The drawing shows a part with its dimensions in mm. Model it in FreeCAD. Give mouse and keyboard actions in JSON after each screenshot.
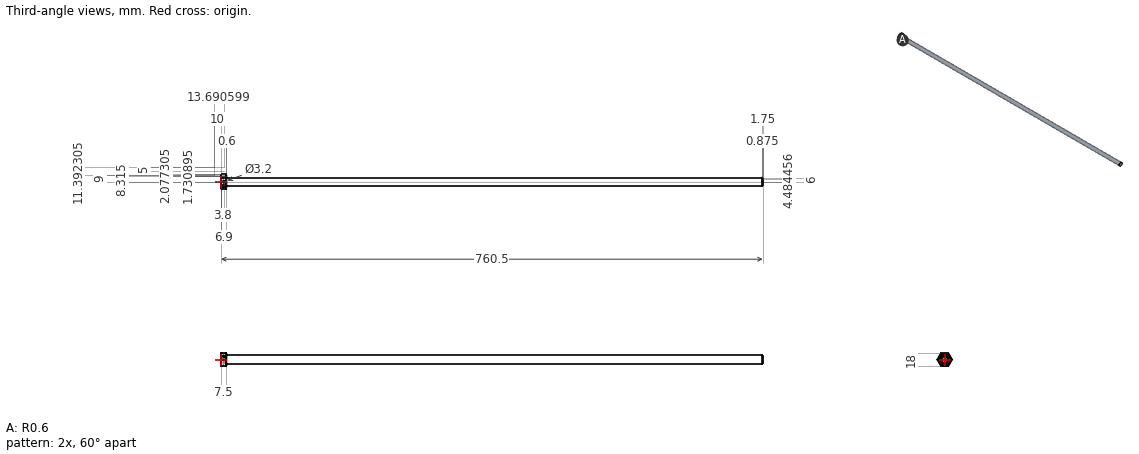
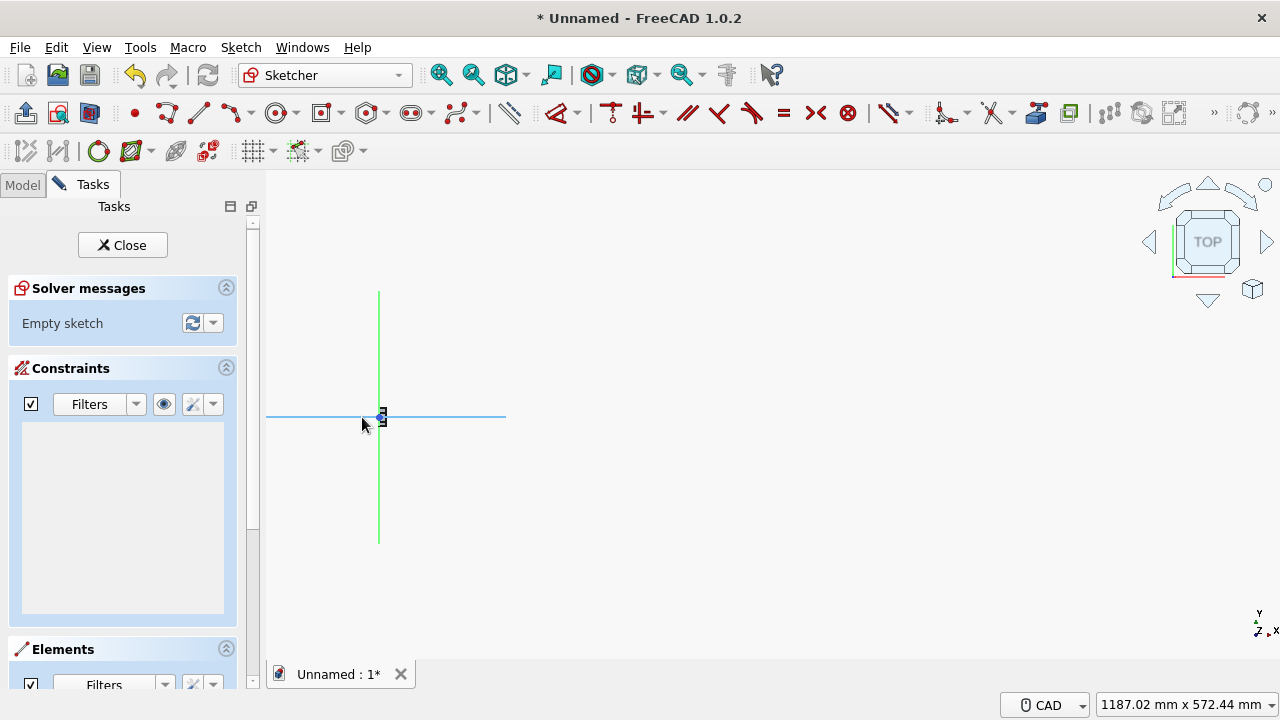
{"action": "key", "text": "g r"}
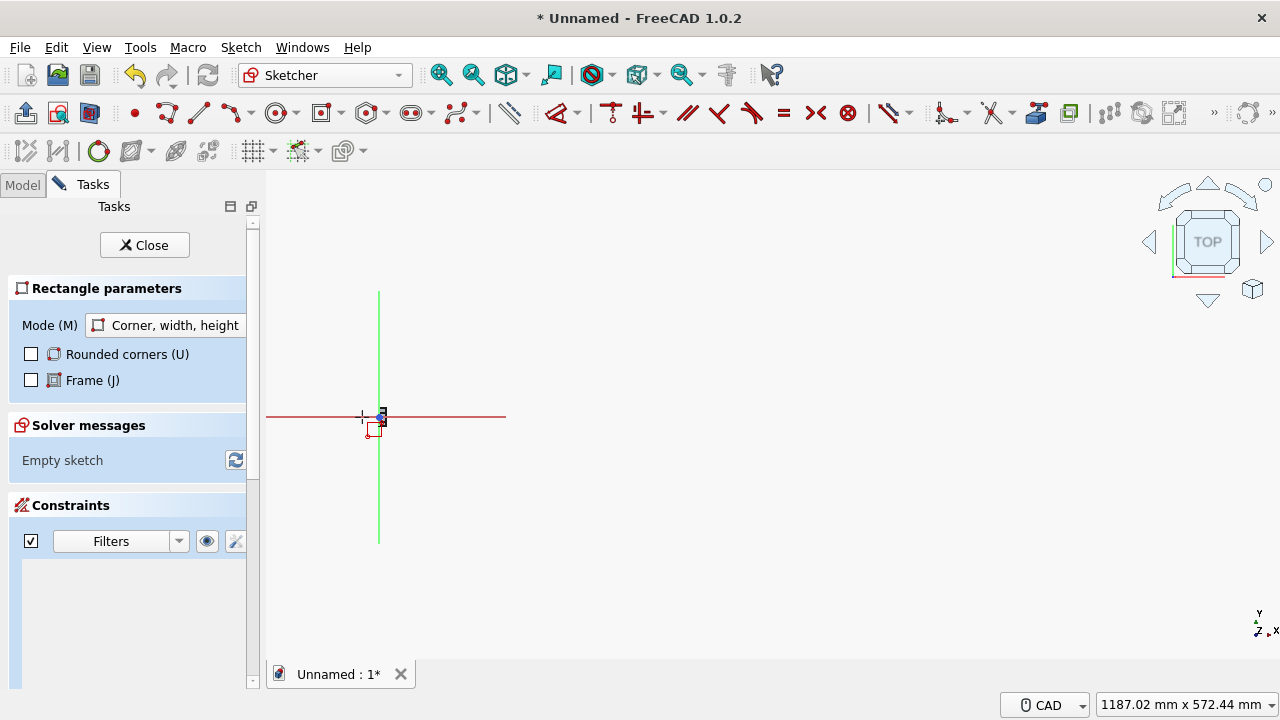
{"action": "scroll", "coordinate": [379, 417], "scroll_direction": "up", "scroll_amount": 6}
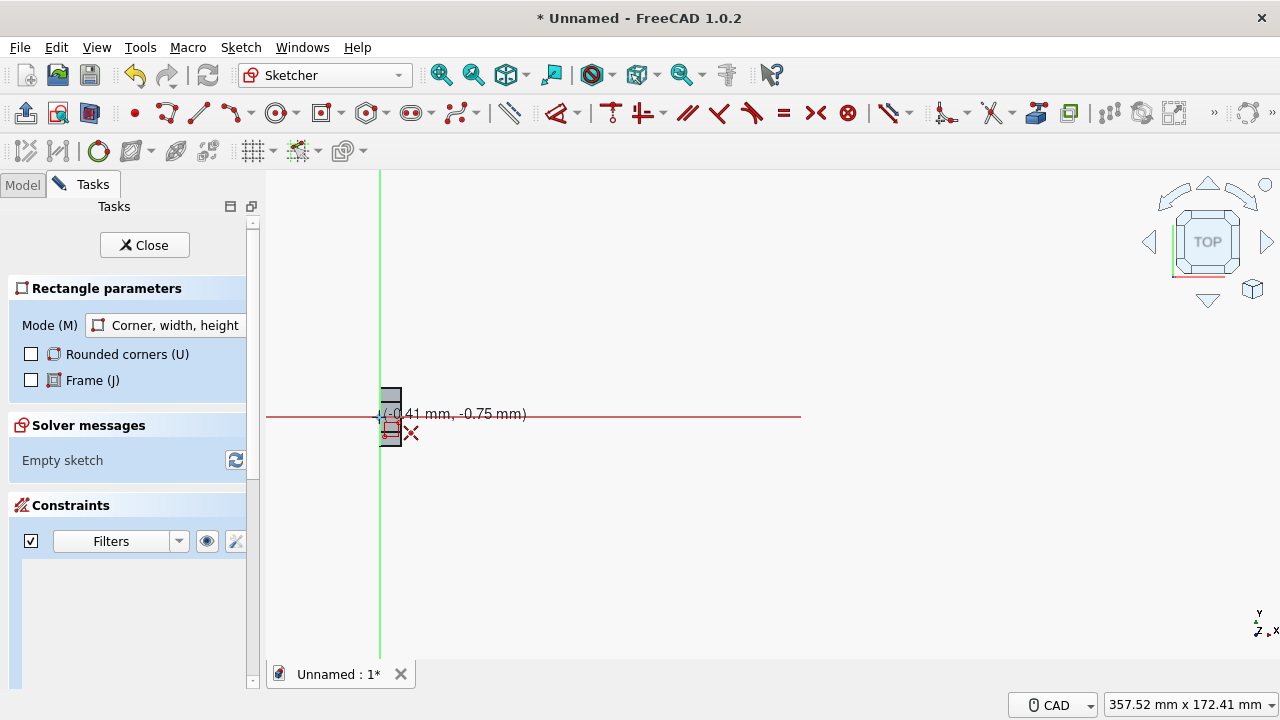
{"action": "left_click", "coordinate": [380, 417]}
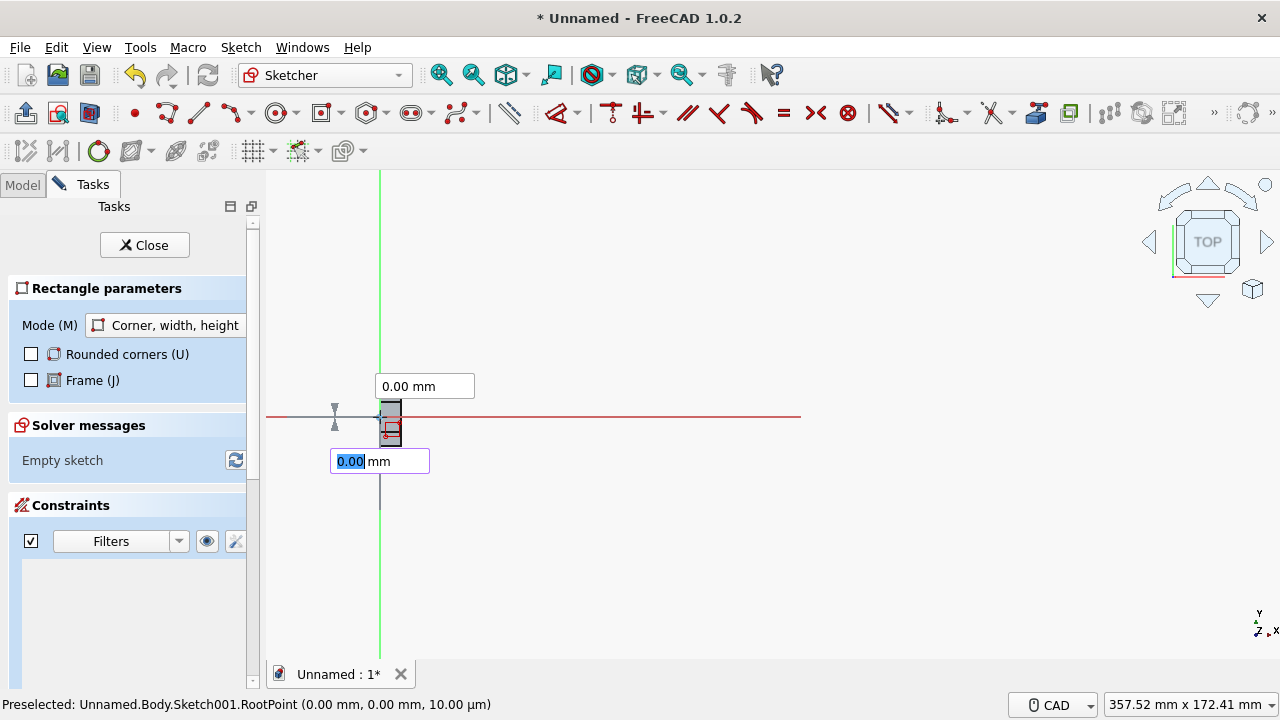
{"action": "scroll", "coordinate": [458, 416], "scroll_direction": "down", "scroll_amount": 7}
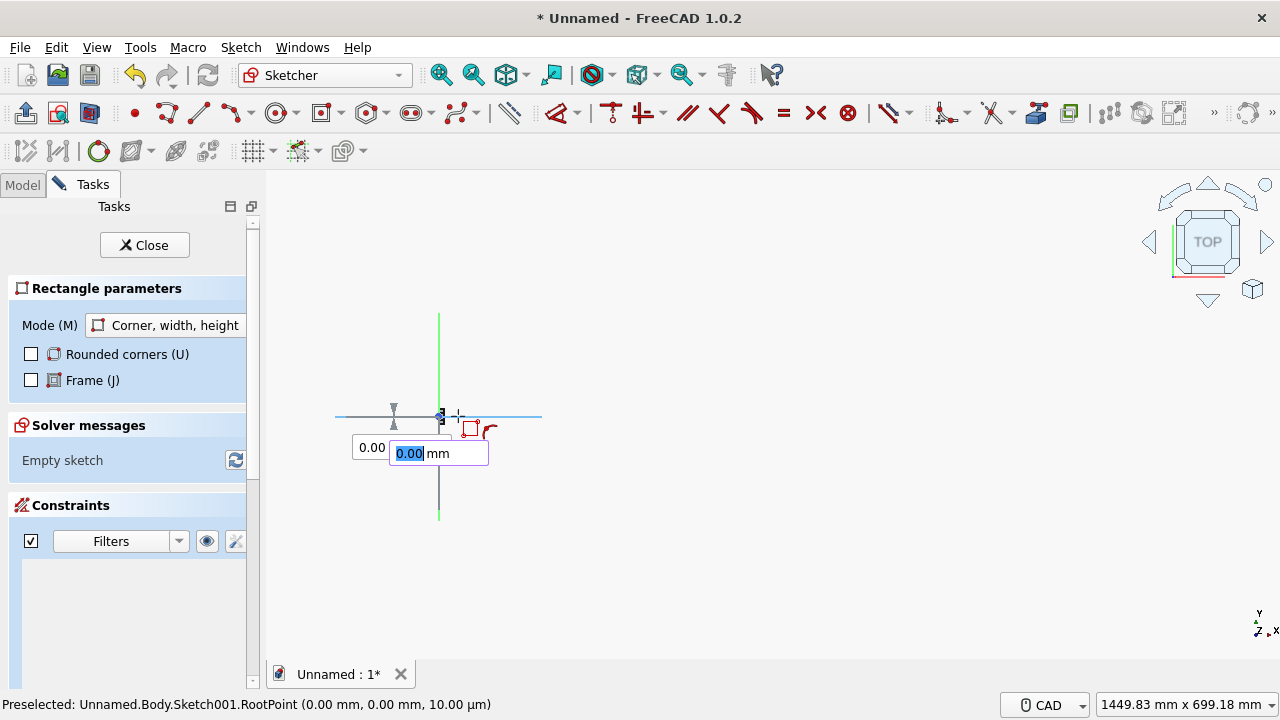
{"action": "scroll", "coordinate": [971, 412], "scroll_direction": "up", "scroll_amount": 7}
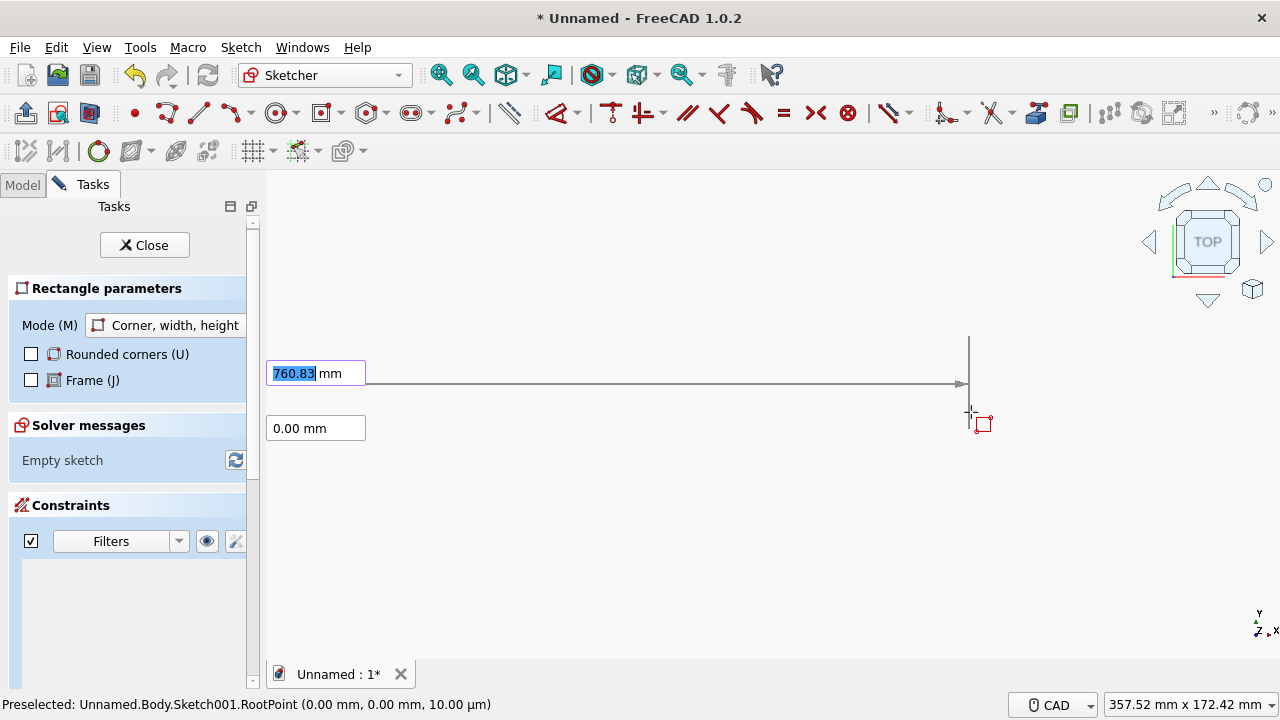
{"action": "left_click", "coordinate": [968, 412]}
{"action": "key", "text": "Escape"}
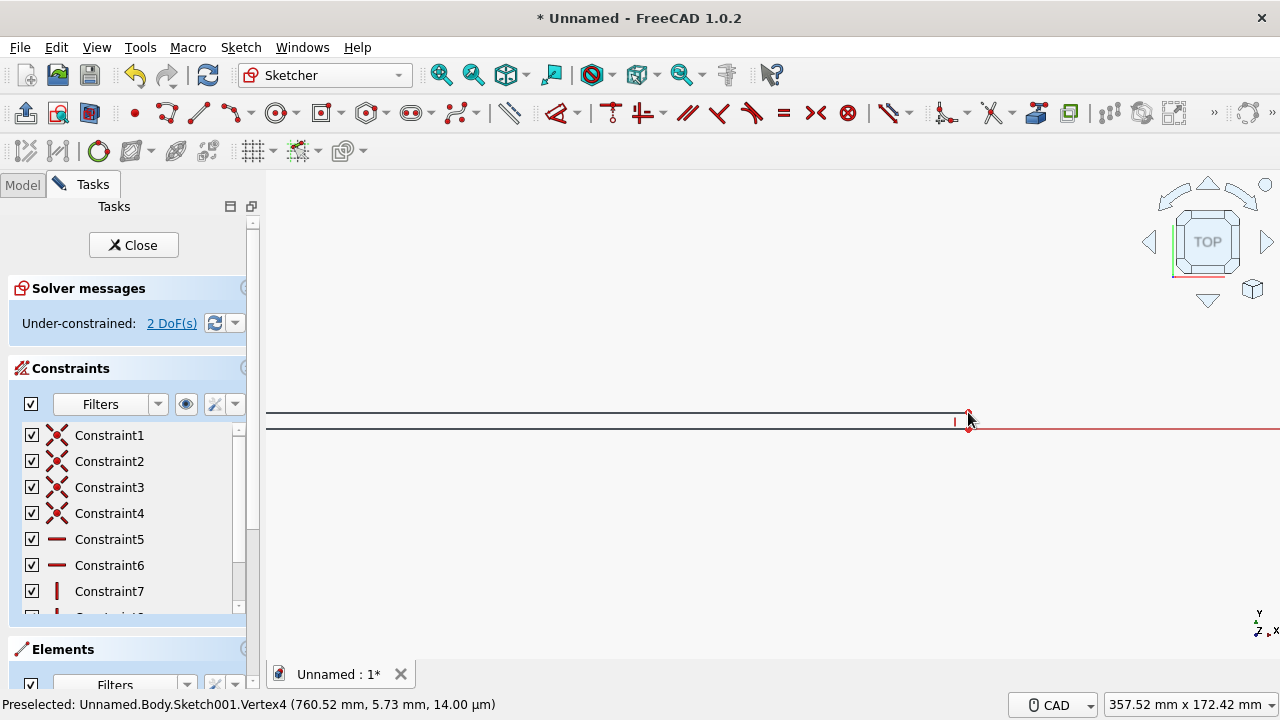
{"action": "key", "text": "d"}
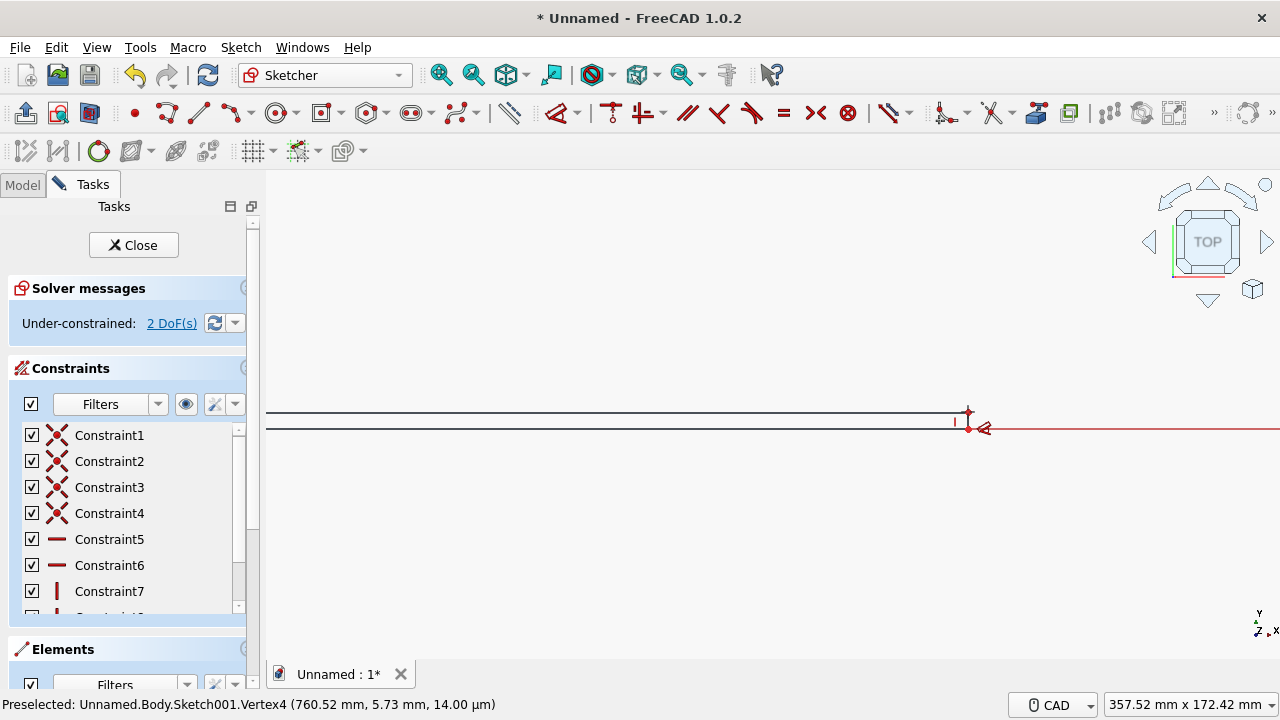
{"action": "scroll", "coordinate": [968, 421], "scroll_direction": "up", "scroll_amount": 5}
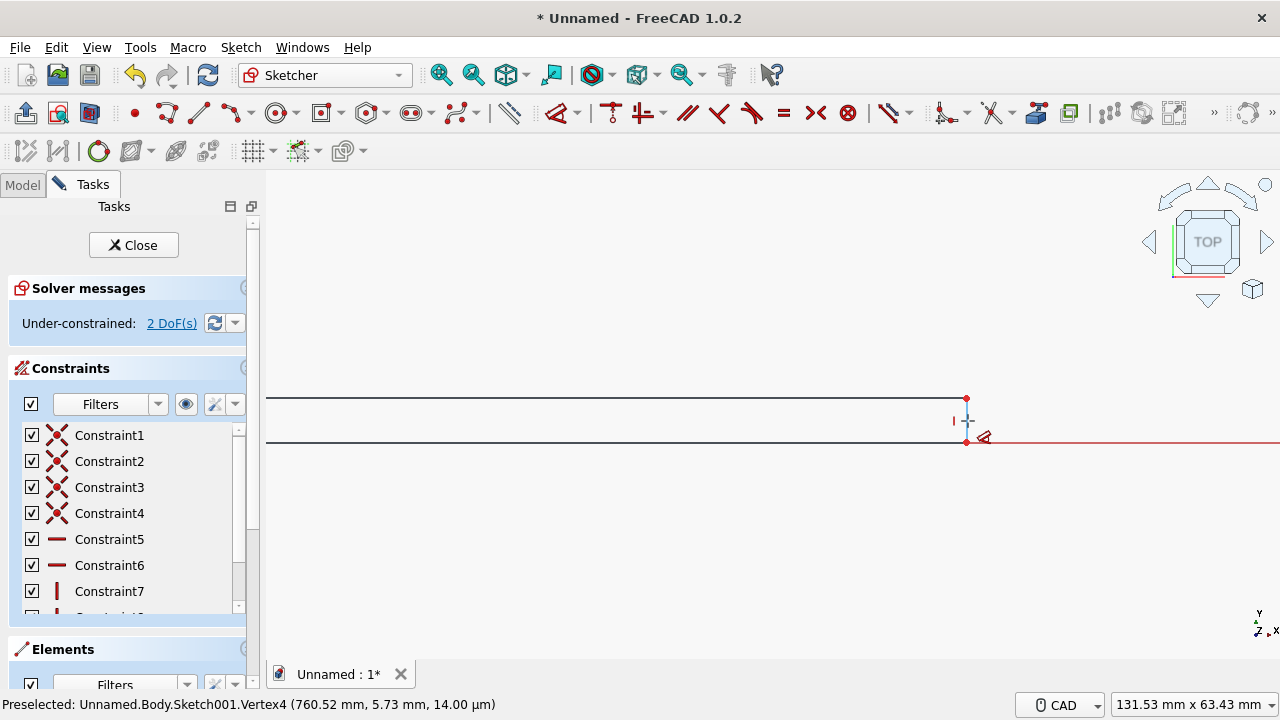
{"action": "left_click", "coordinate": [967, 420]}
{"action": "left_click", "coordinate": [1001, 420]}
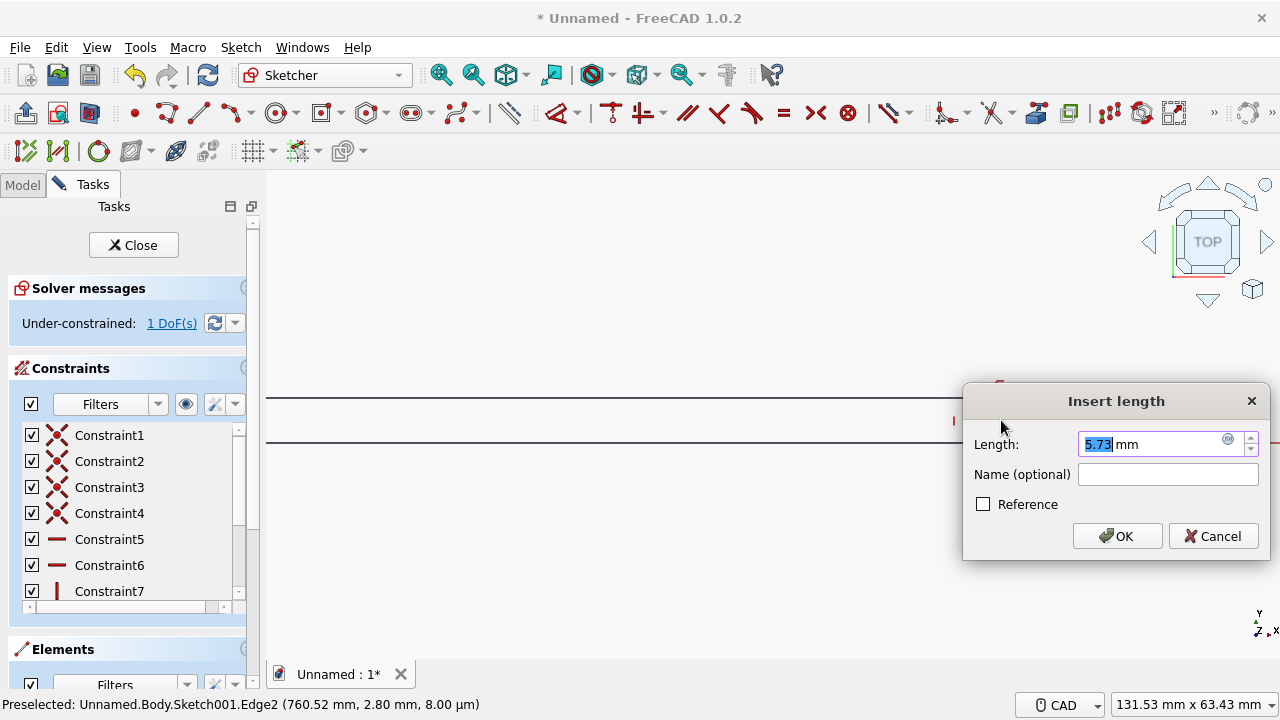
{"action": "type", "text": "6"}
{"action": "key", "text": "Return"}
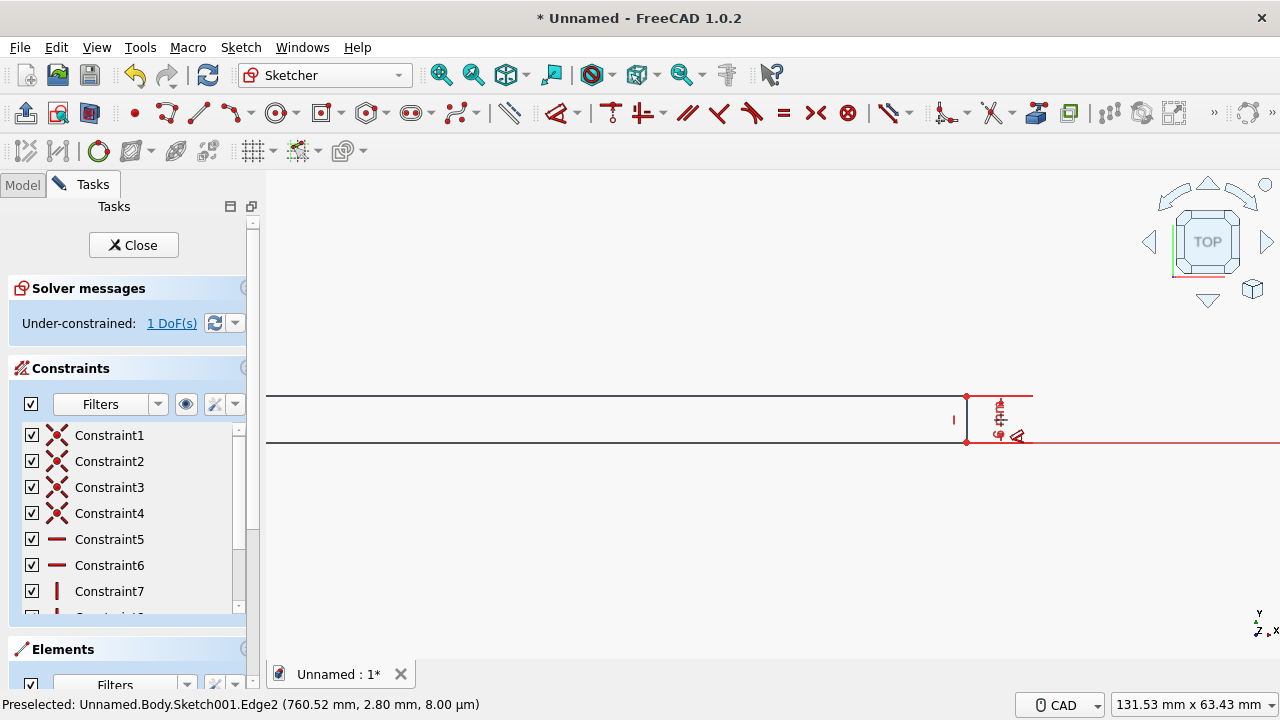
{"action": "scroll", "coordinate": [971, 414], "scroll_direction": "down", "scroll_amount": 12}